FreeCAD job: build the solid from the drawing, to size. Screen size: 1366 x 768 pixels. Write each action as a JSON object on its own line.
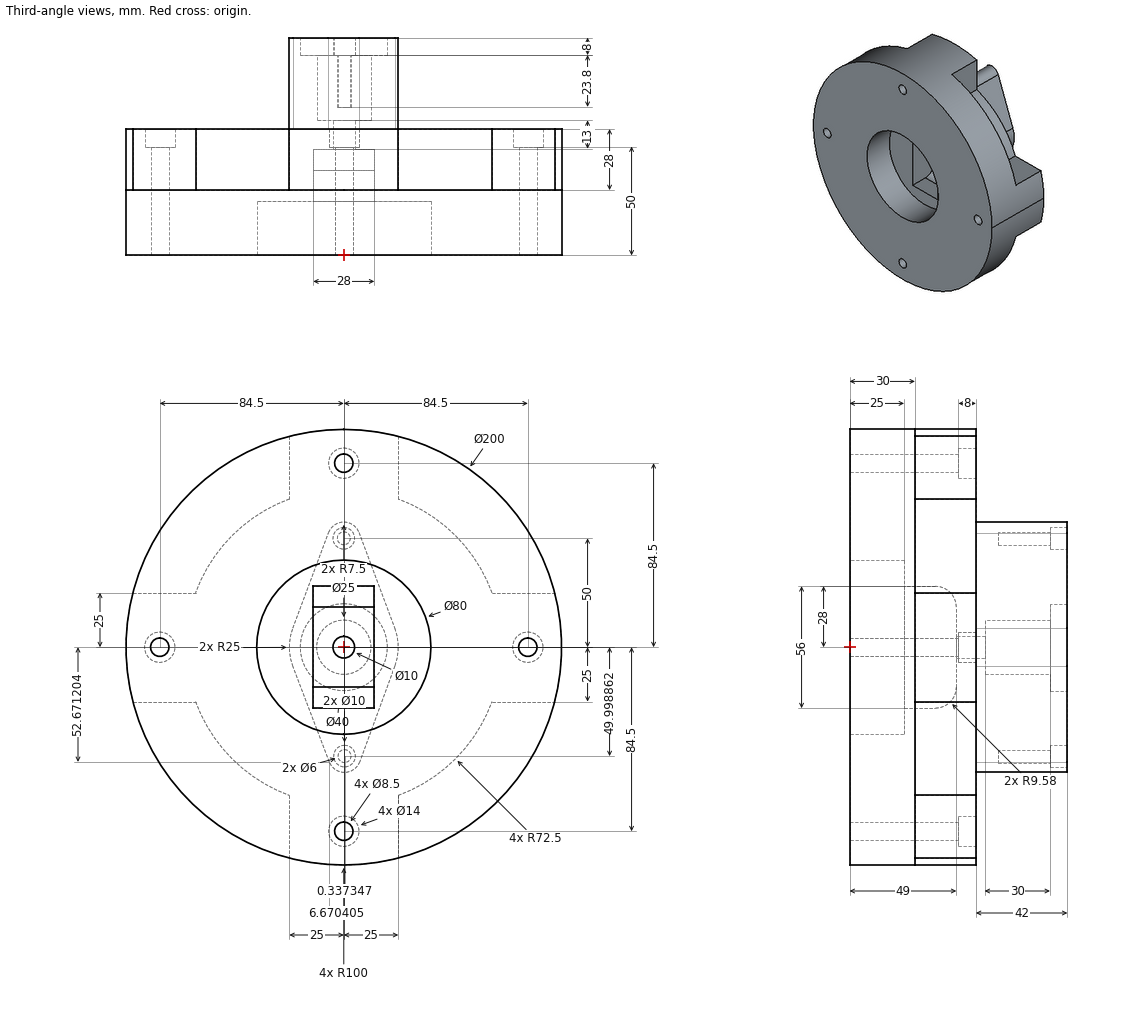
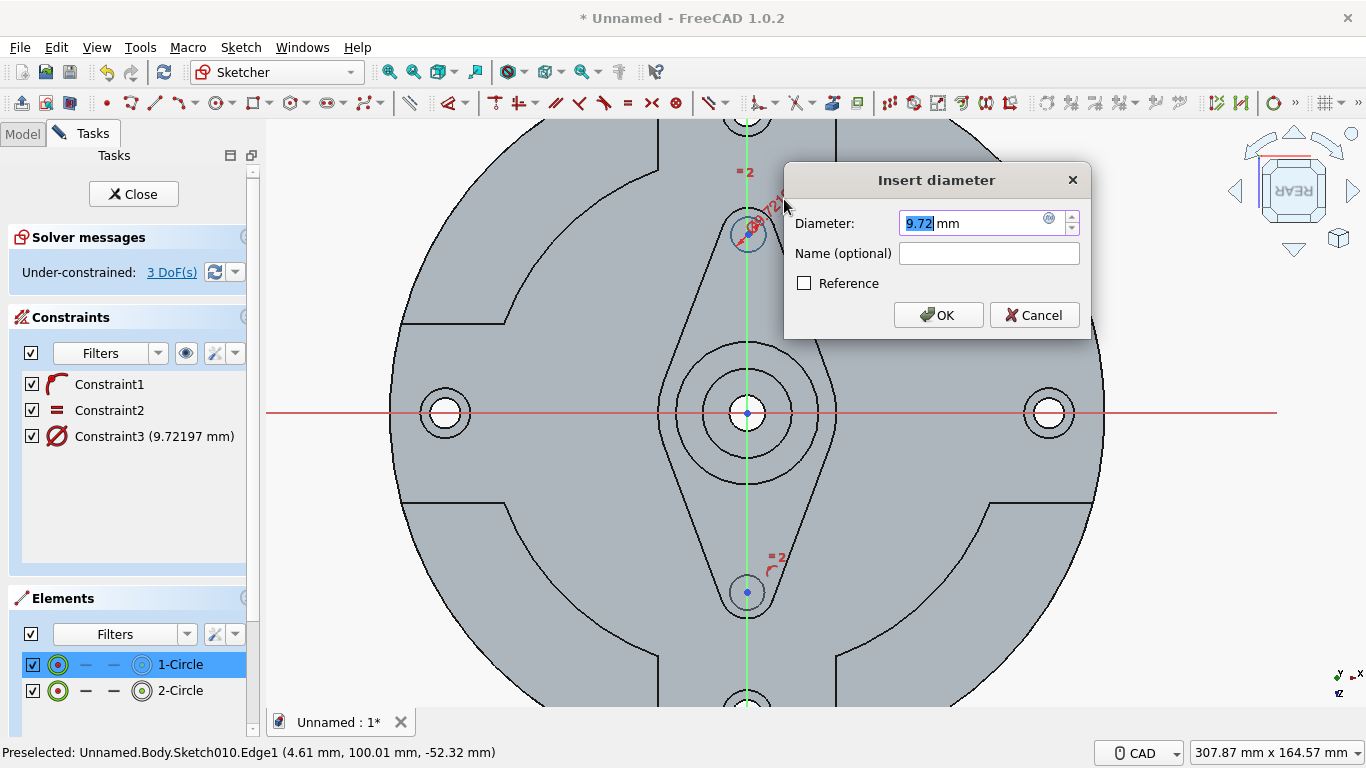
{"action": "type", "text": "10"}
{"action": "key", "text": "Return"}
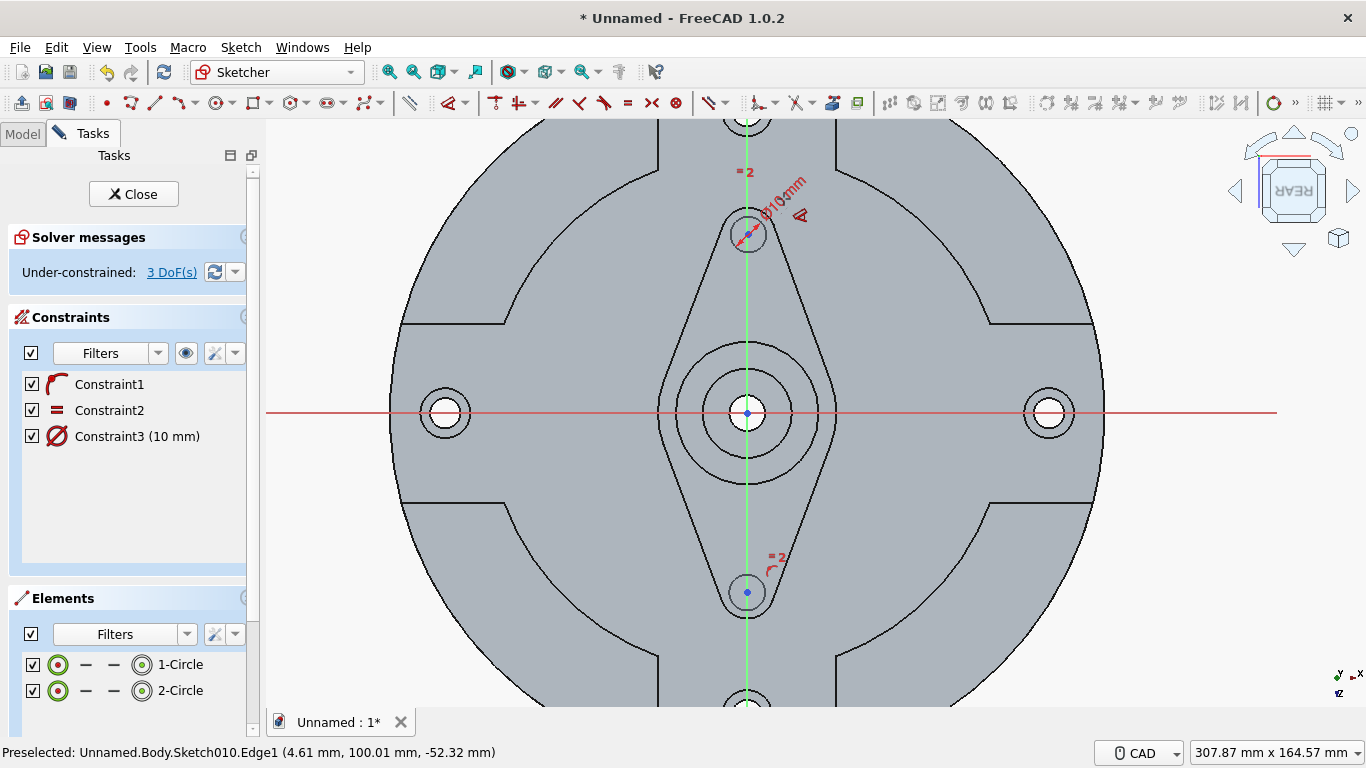
{"action": "left_click", "coordinate": [747, 593]}
{"action": "left_click", "coordinate": [713, 503]}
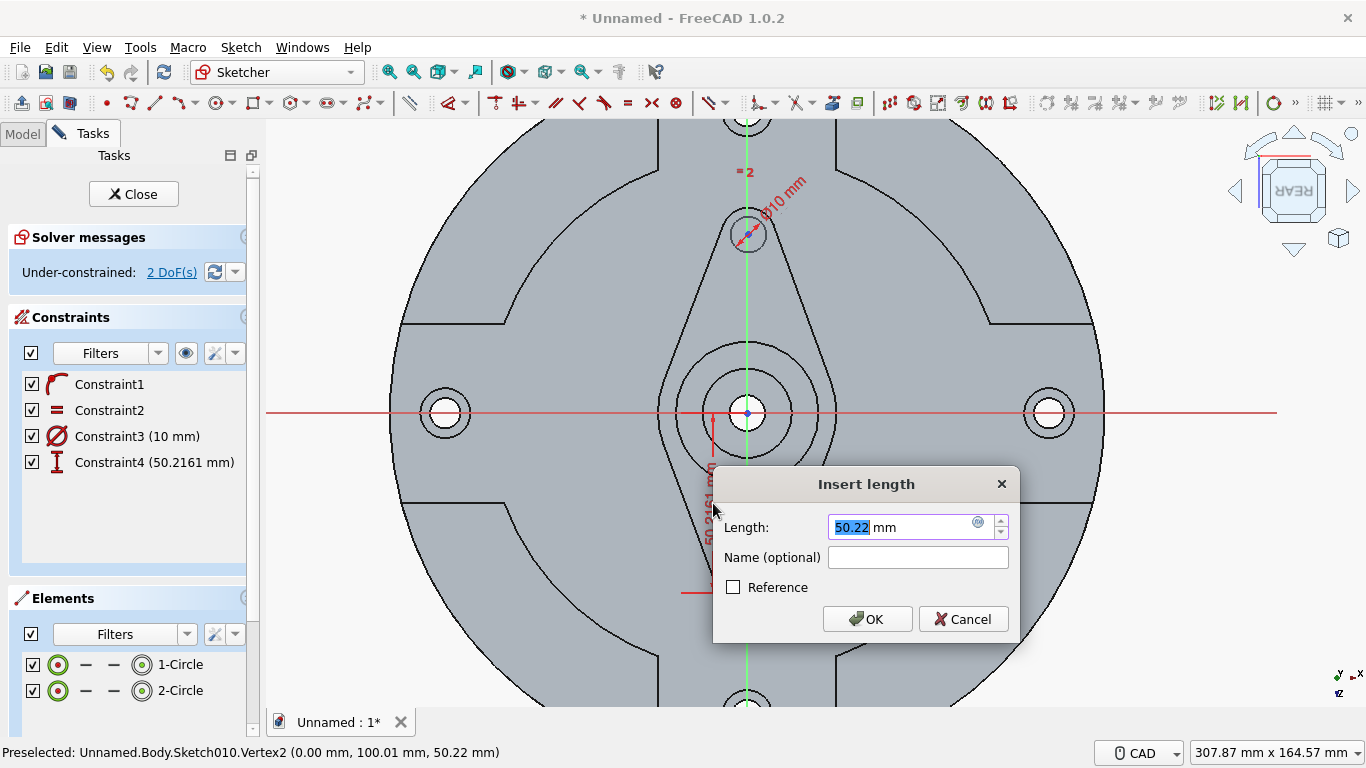
{"action": "type", "text": "50"}
{"action": "key", "text": "Return"}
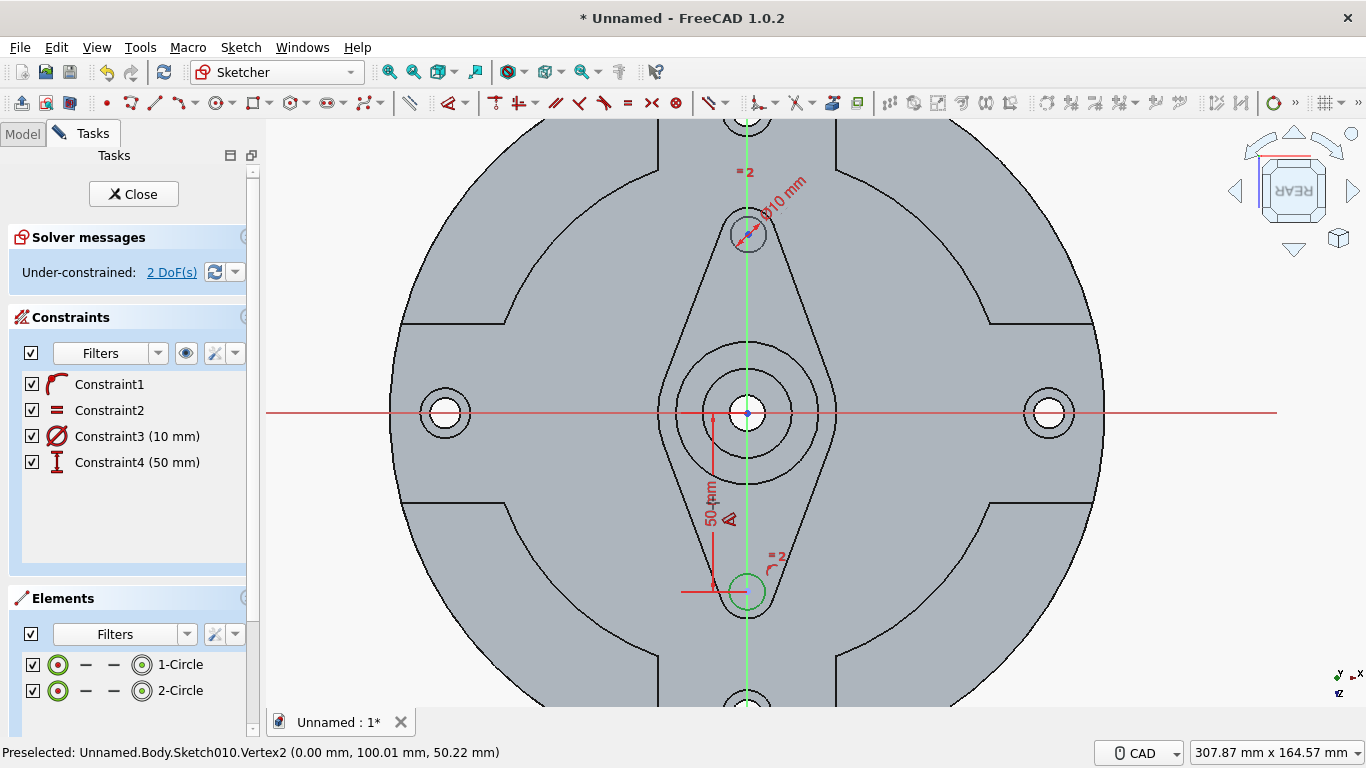
{"action": "scroll", "coordinate": [748, 235], "scroll_direction": "up", "scroll_amount": 18}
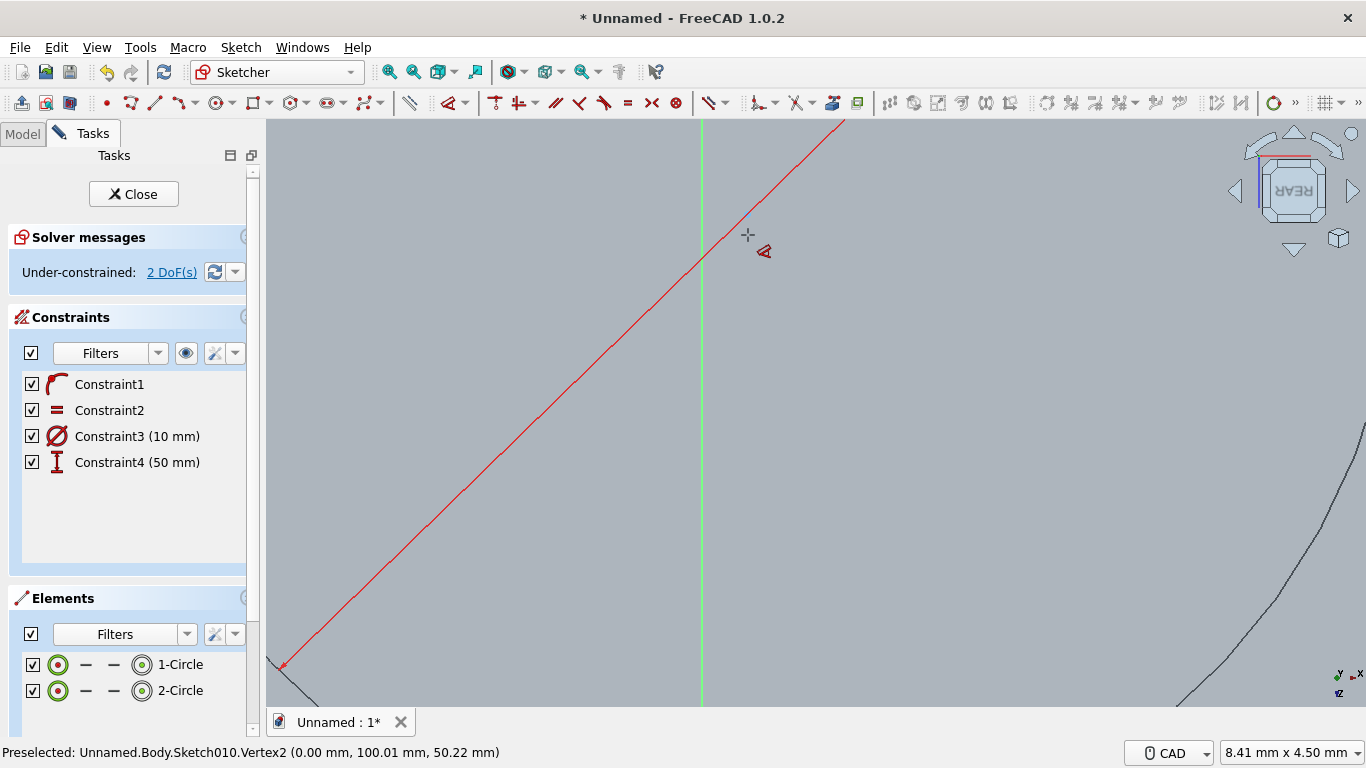
{"action": "left_click", "coordinate": [747, 214]}
{"action": "left_click", "coordinate": [725, 180]}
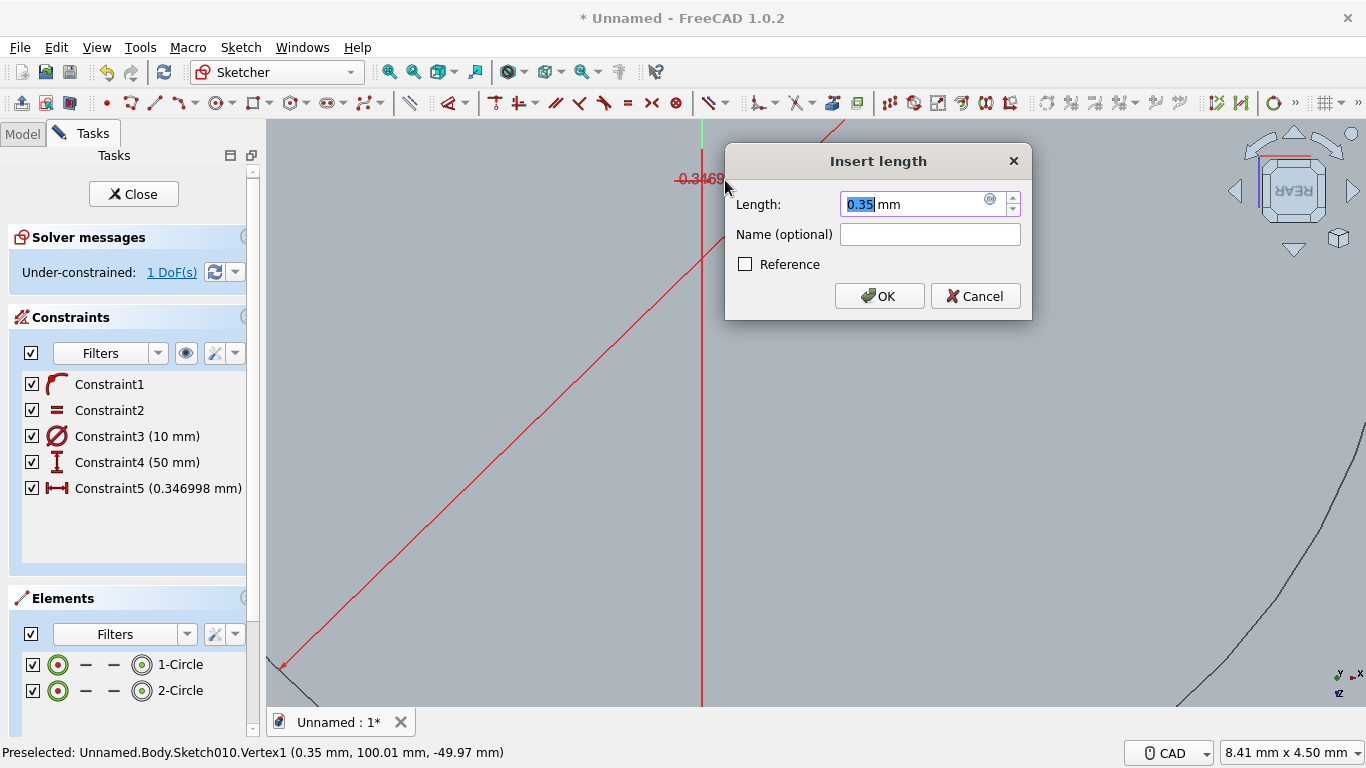
{"action": "type", "text": "0.337347"}
{"action": "key", "text": "Return"}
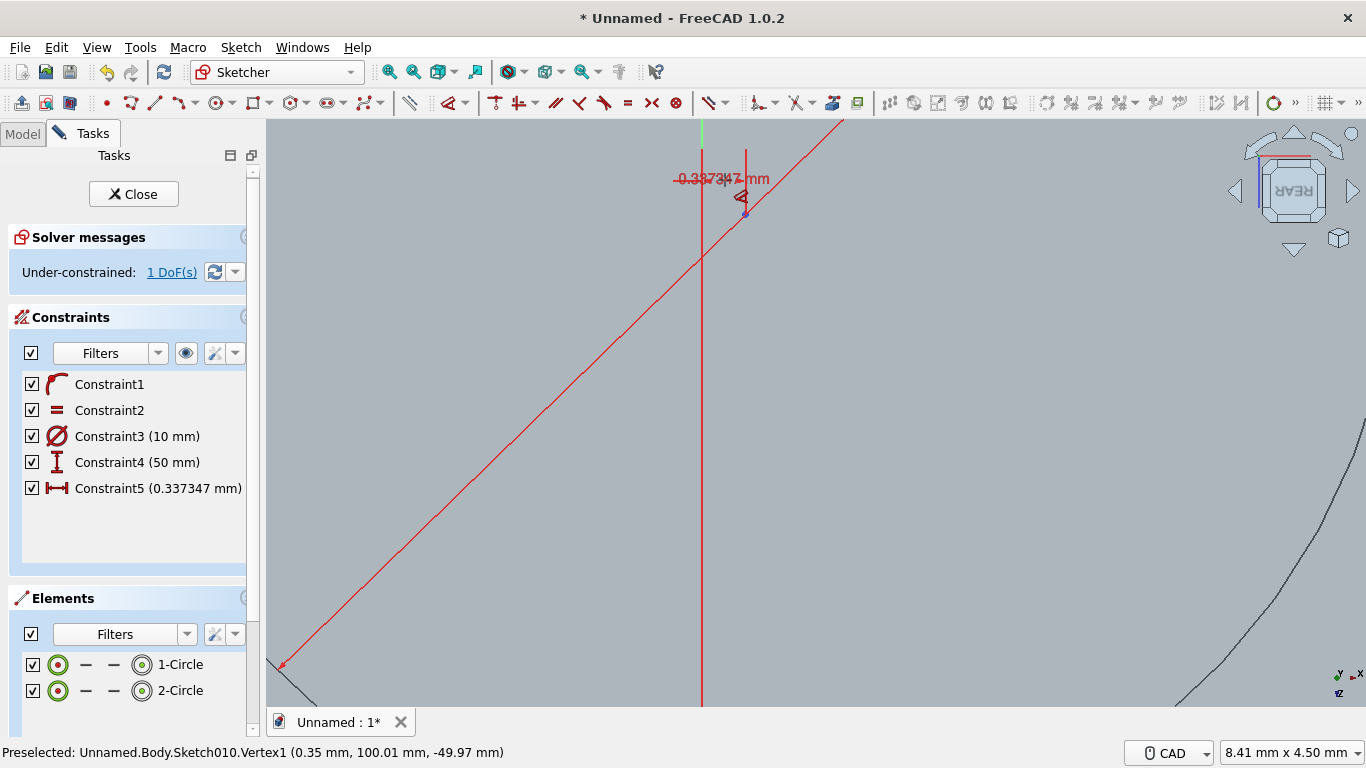
{"action": "scroll", "coordinate": [748, 194], "scroll_direction": "down", "scroll_amount": 17}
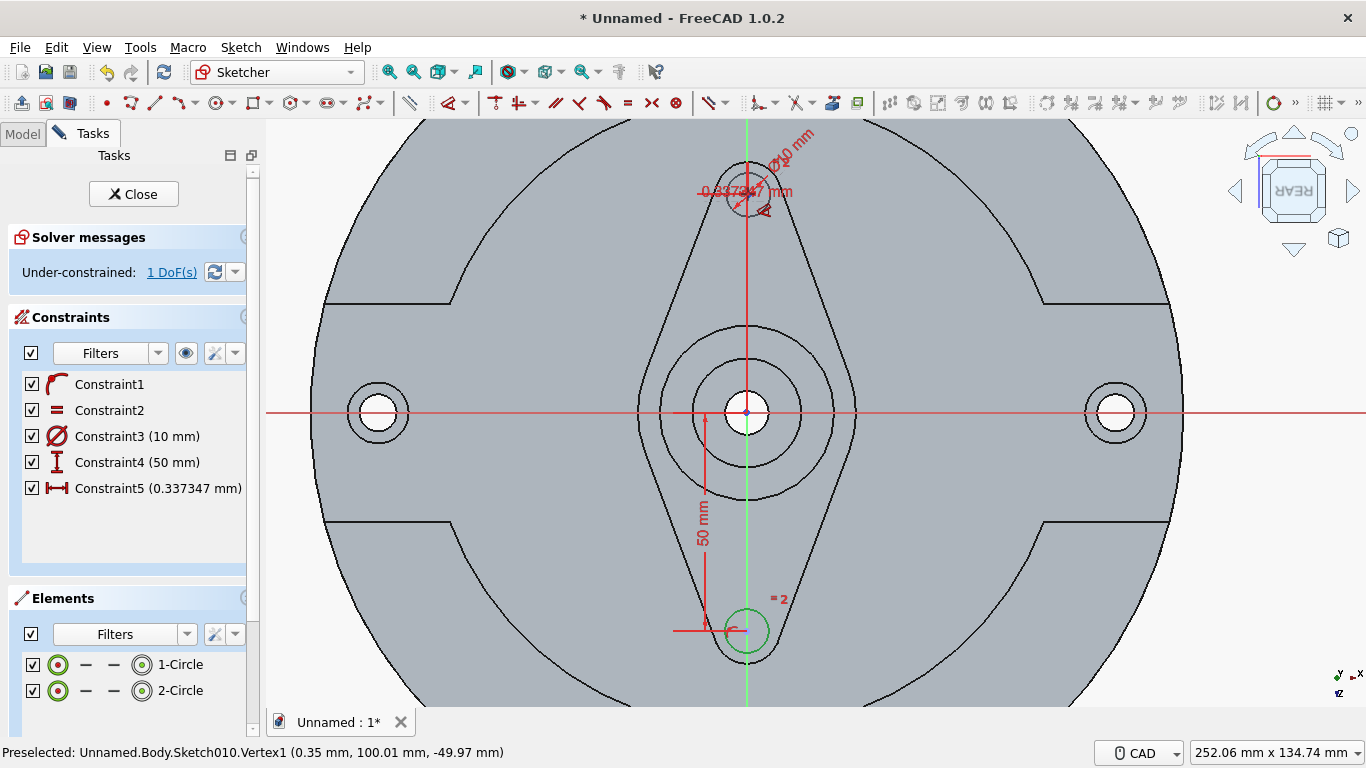
{"action": "left_click", "coordinate": [748, 195]}
{"action": "left_click", "coordinate": [713, 304]}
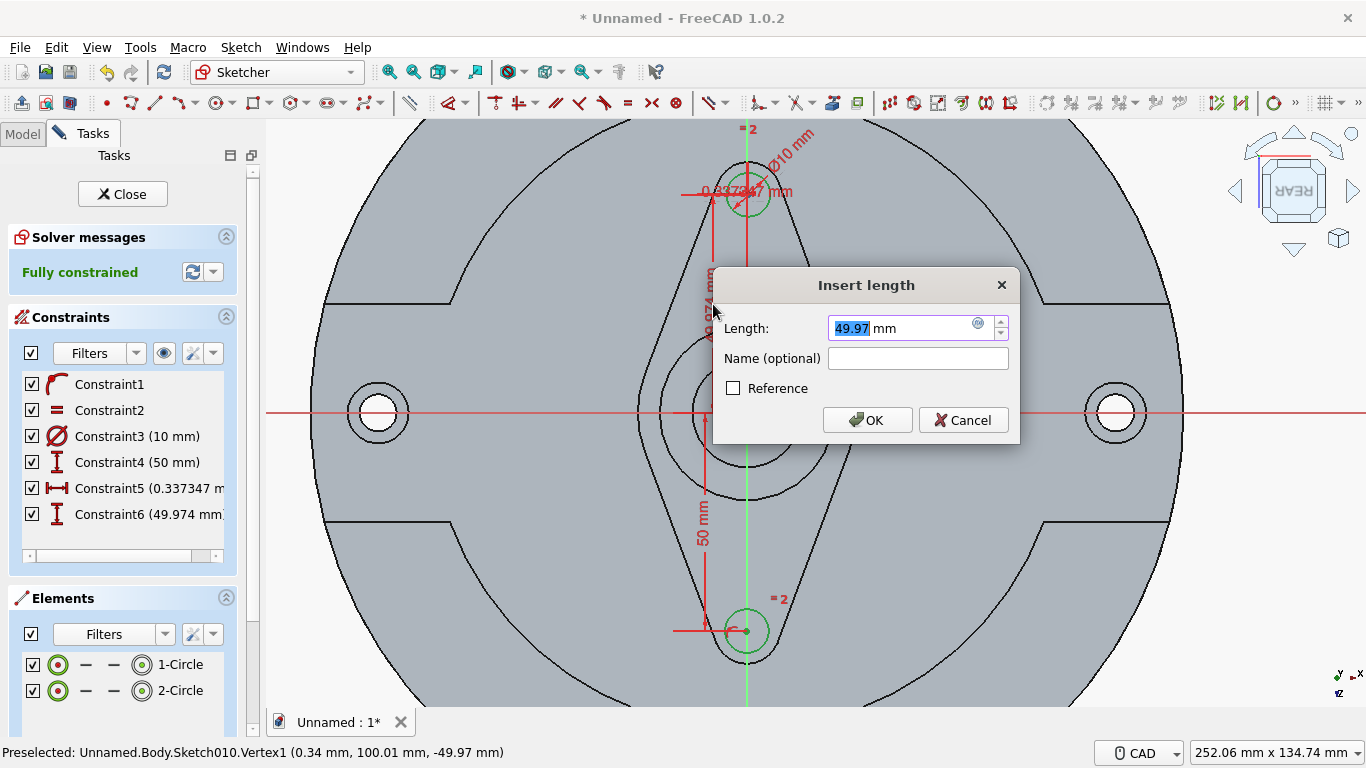
{"action": "type", "text": "49.998862"}
{"action": "key", "text": "Return"}
{"action": "key", "text": "Escape"}